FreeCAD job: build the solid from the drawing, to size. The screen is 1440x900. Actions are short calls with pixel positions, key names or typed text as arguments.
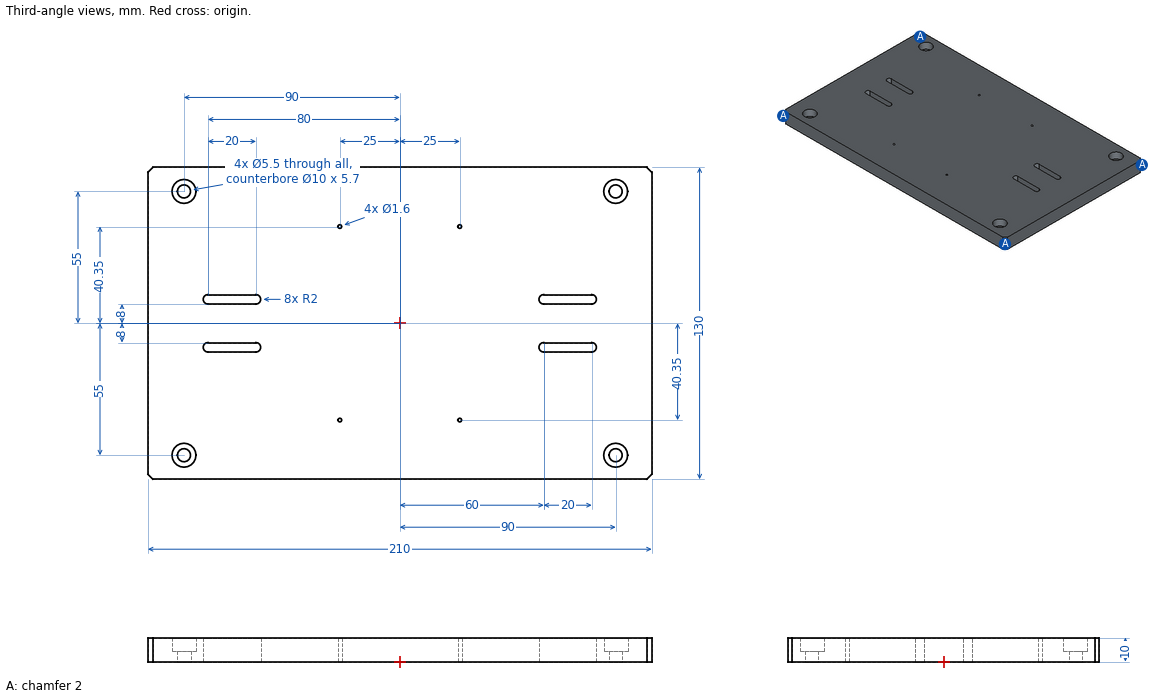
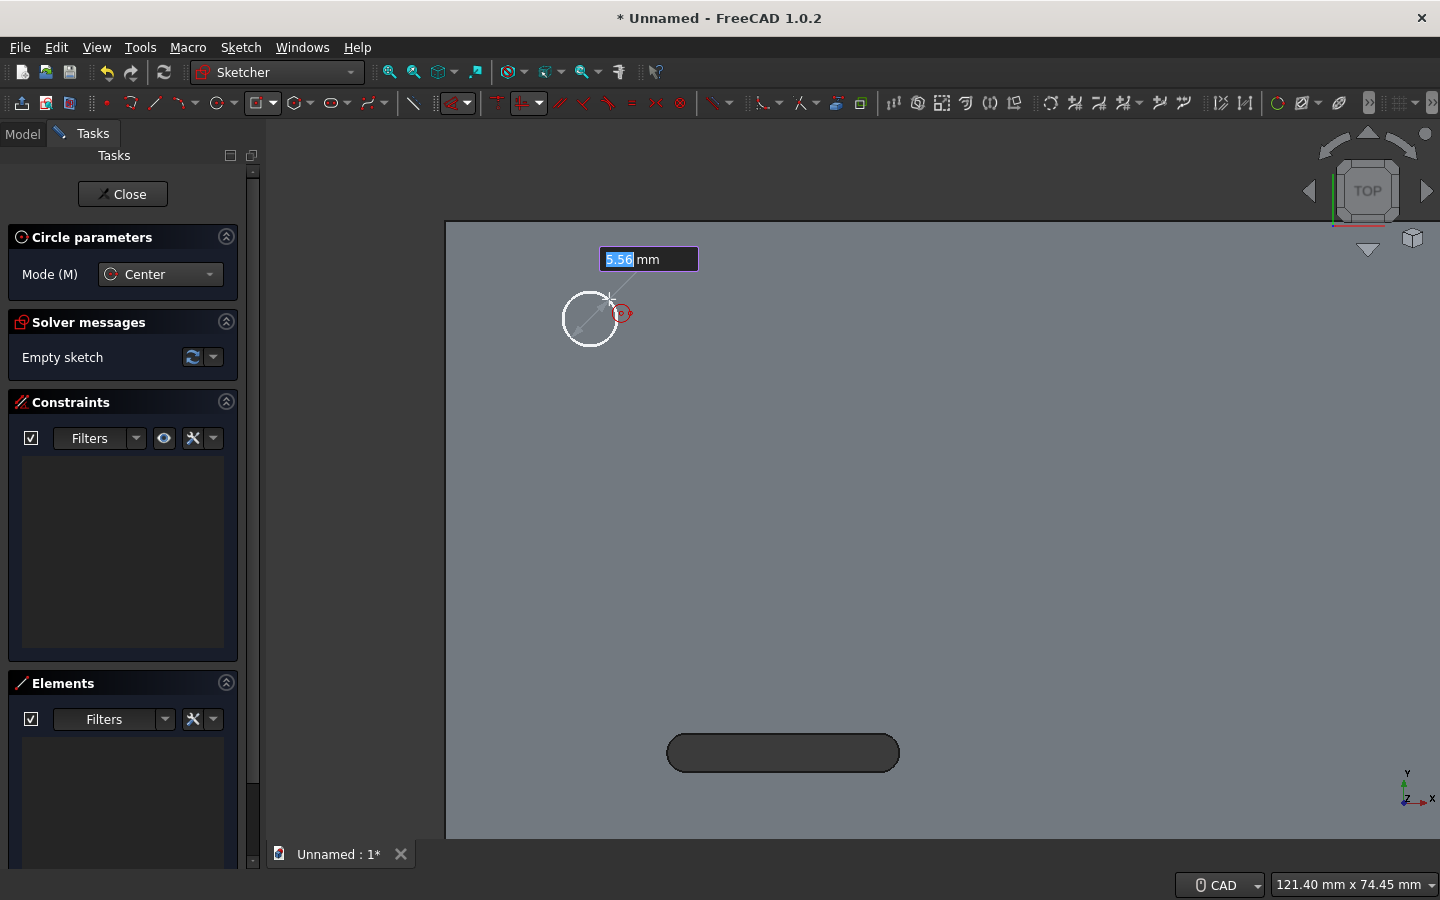
text(5.5)
key(Return)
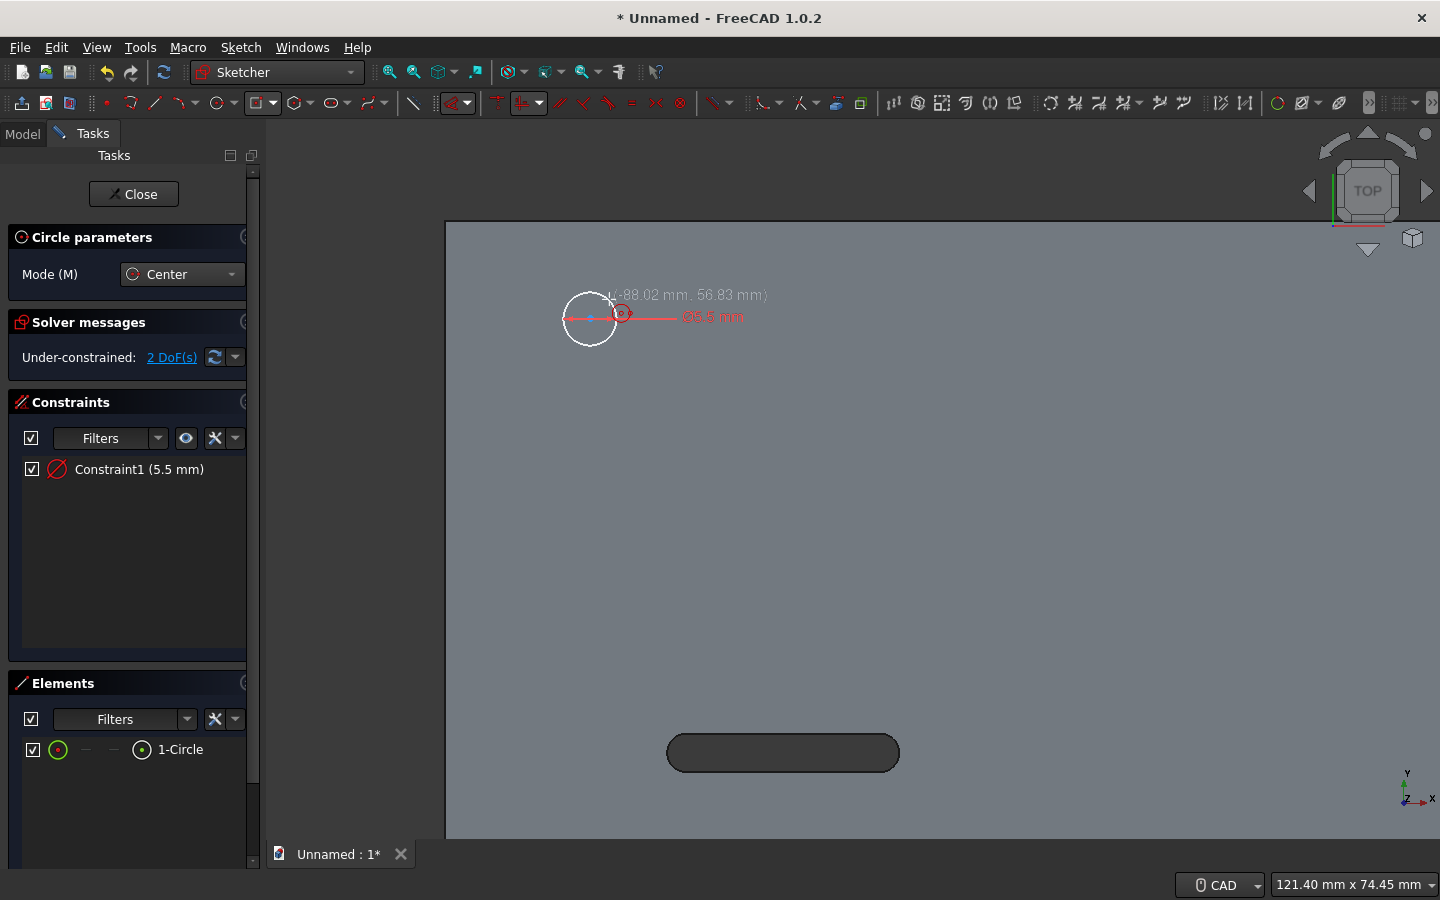
scroll(391, 263, down, 5)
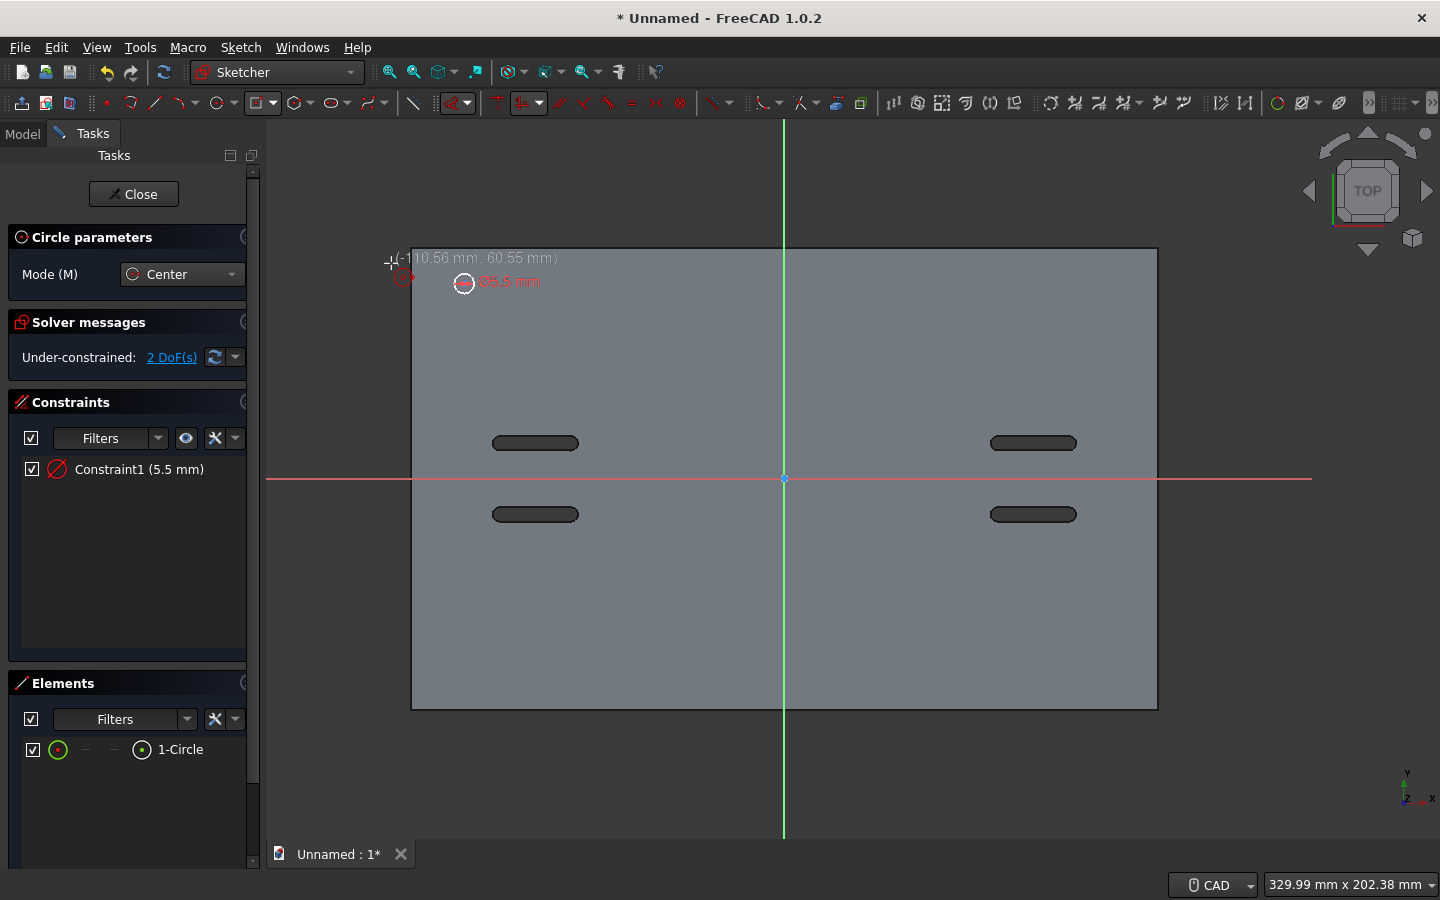
scroll(464, 675, up, 5)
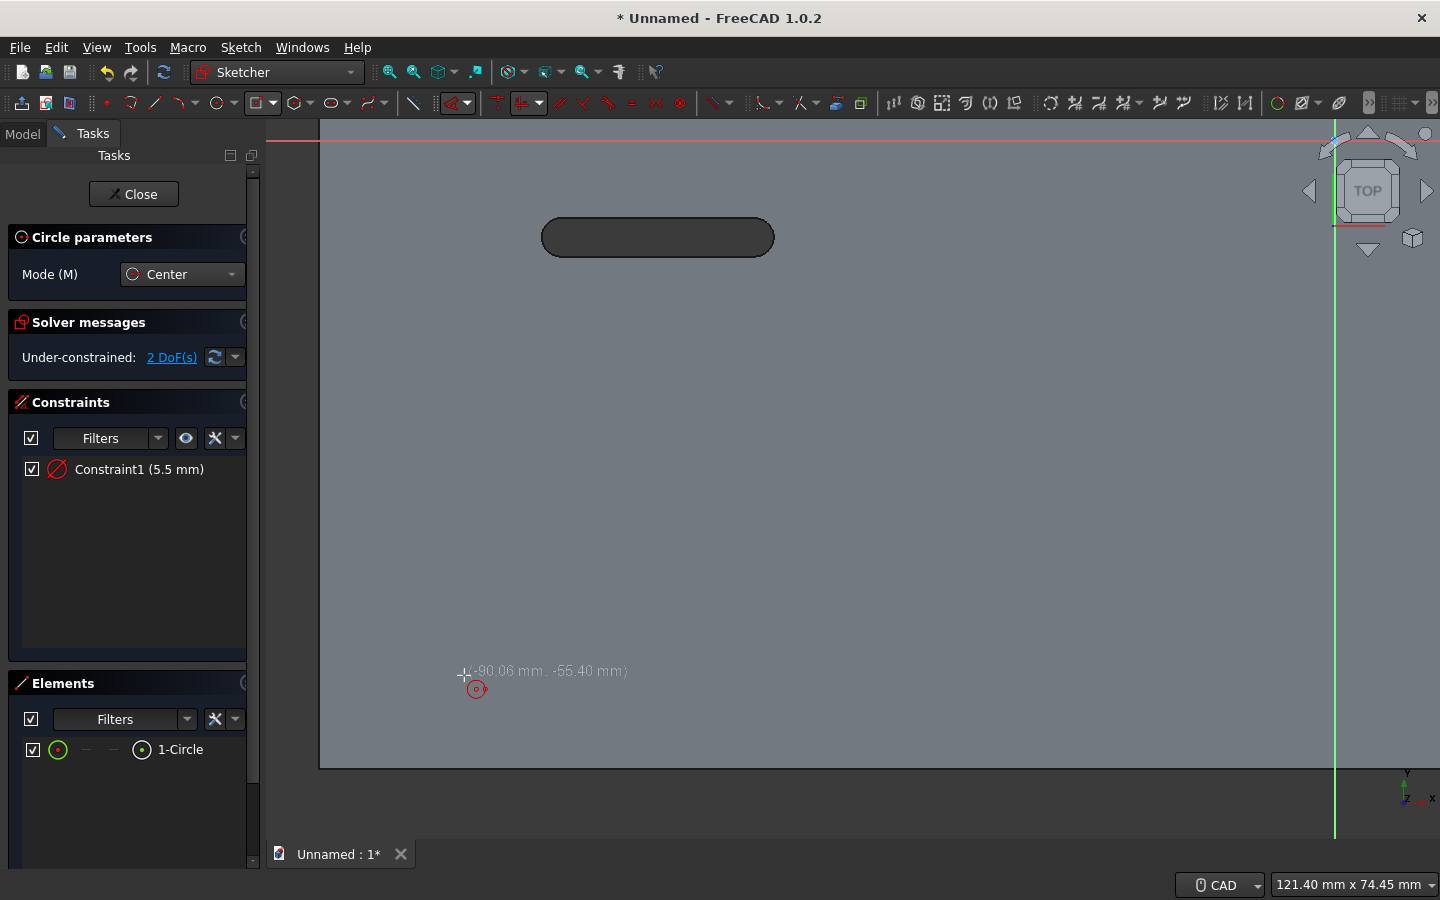
click(464, 673)
move(483, 654)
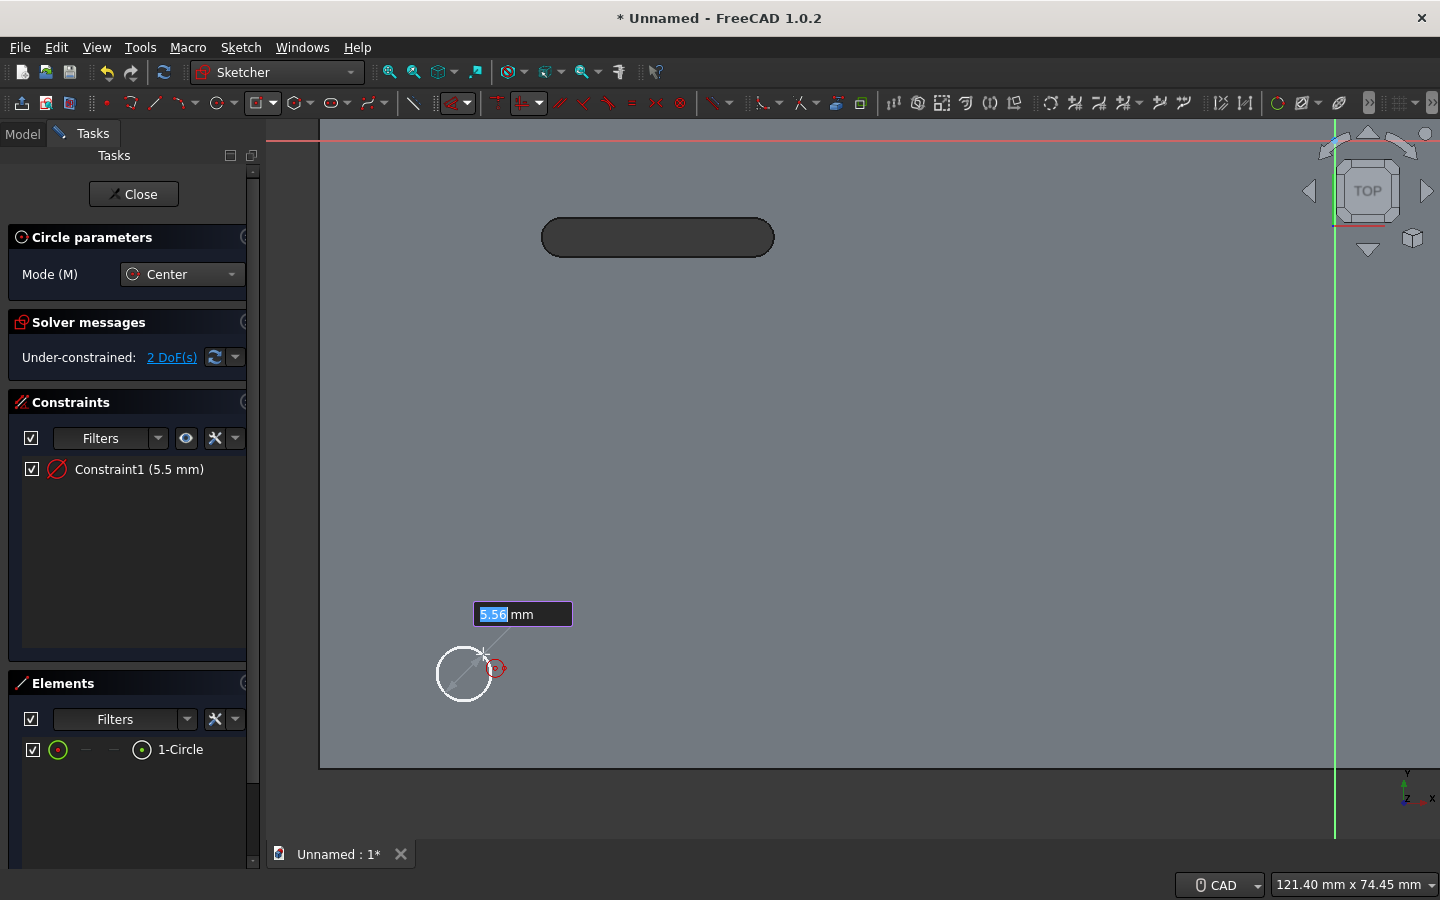
text(5.5)
key(Return)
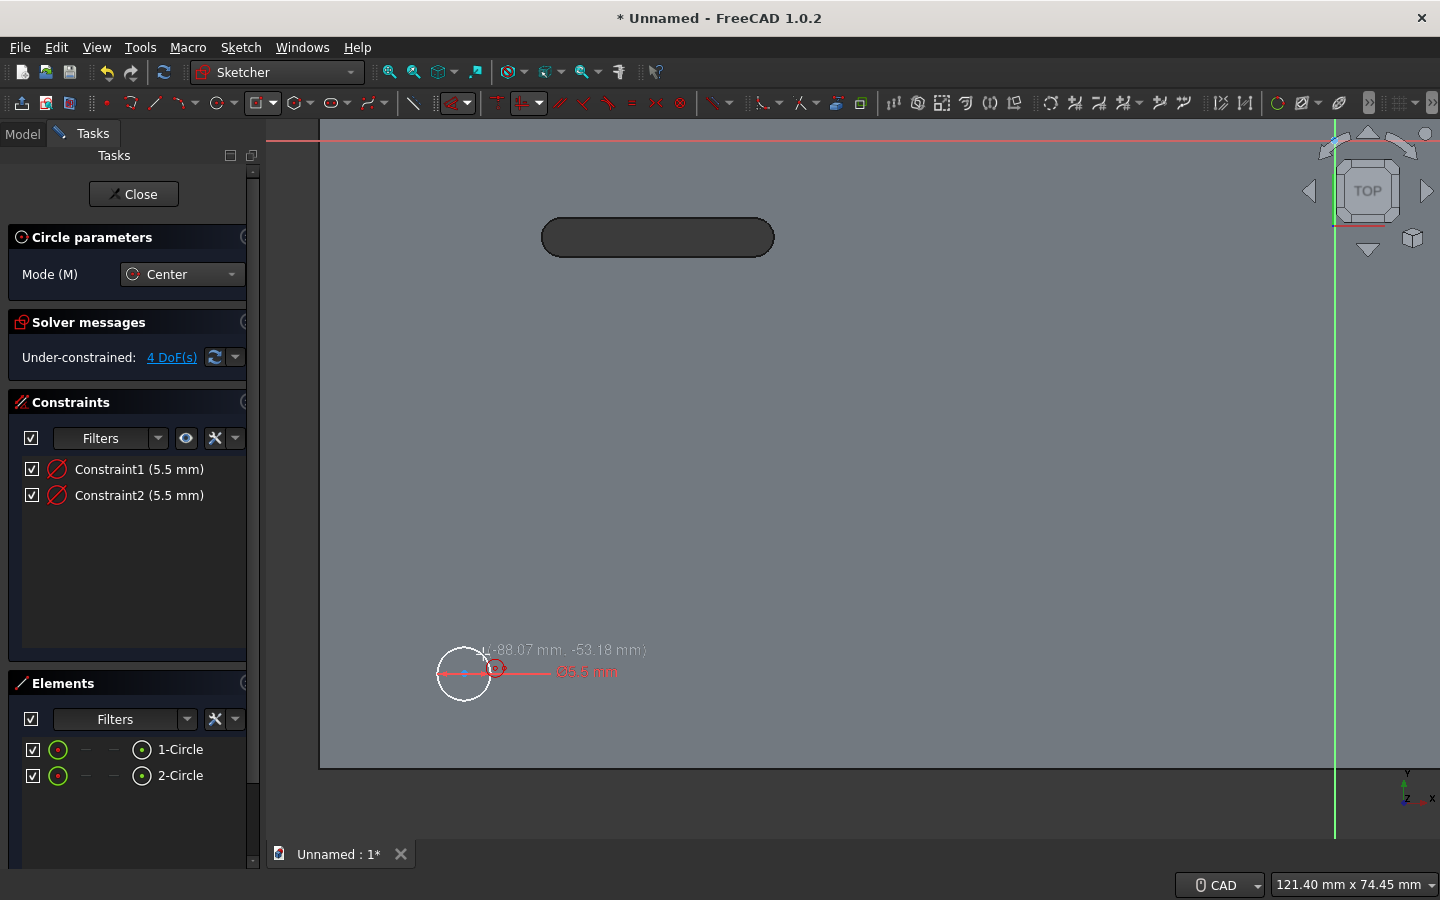
scroll(464, 676, down, 5)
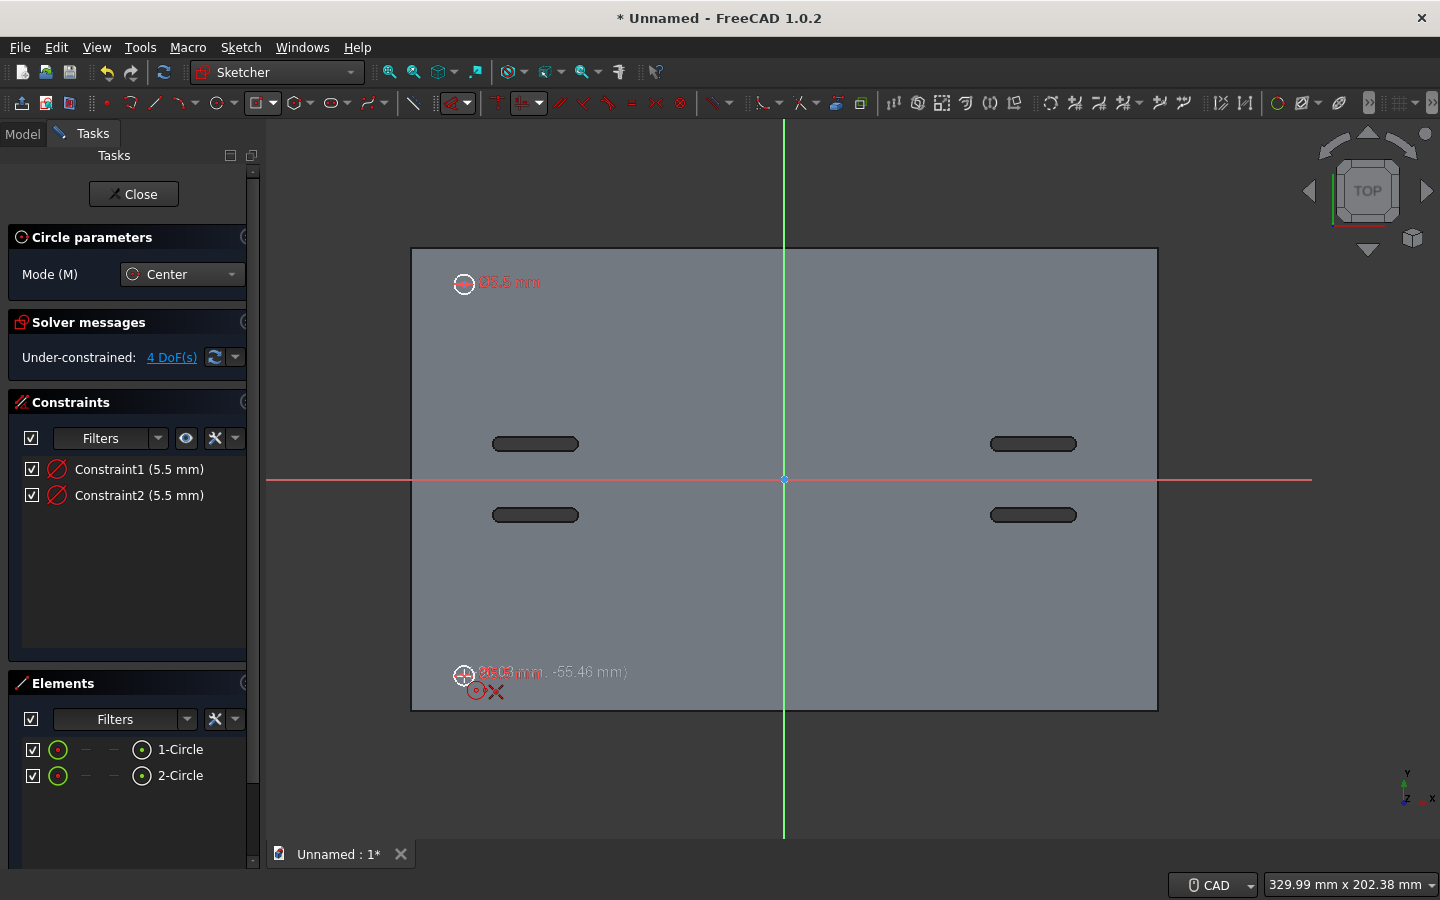
scroll(1105, 675, up, 5)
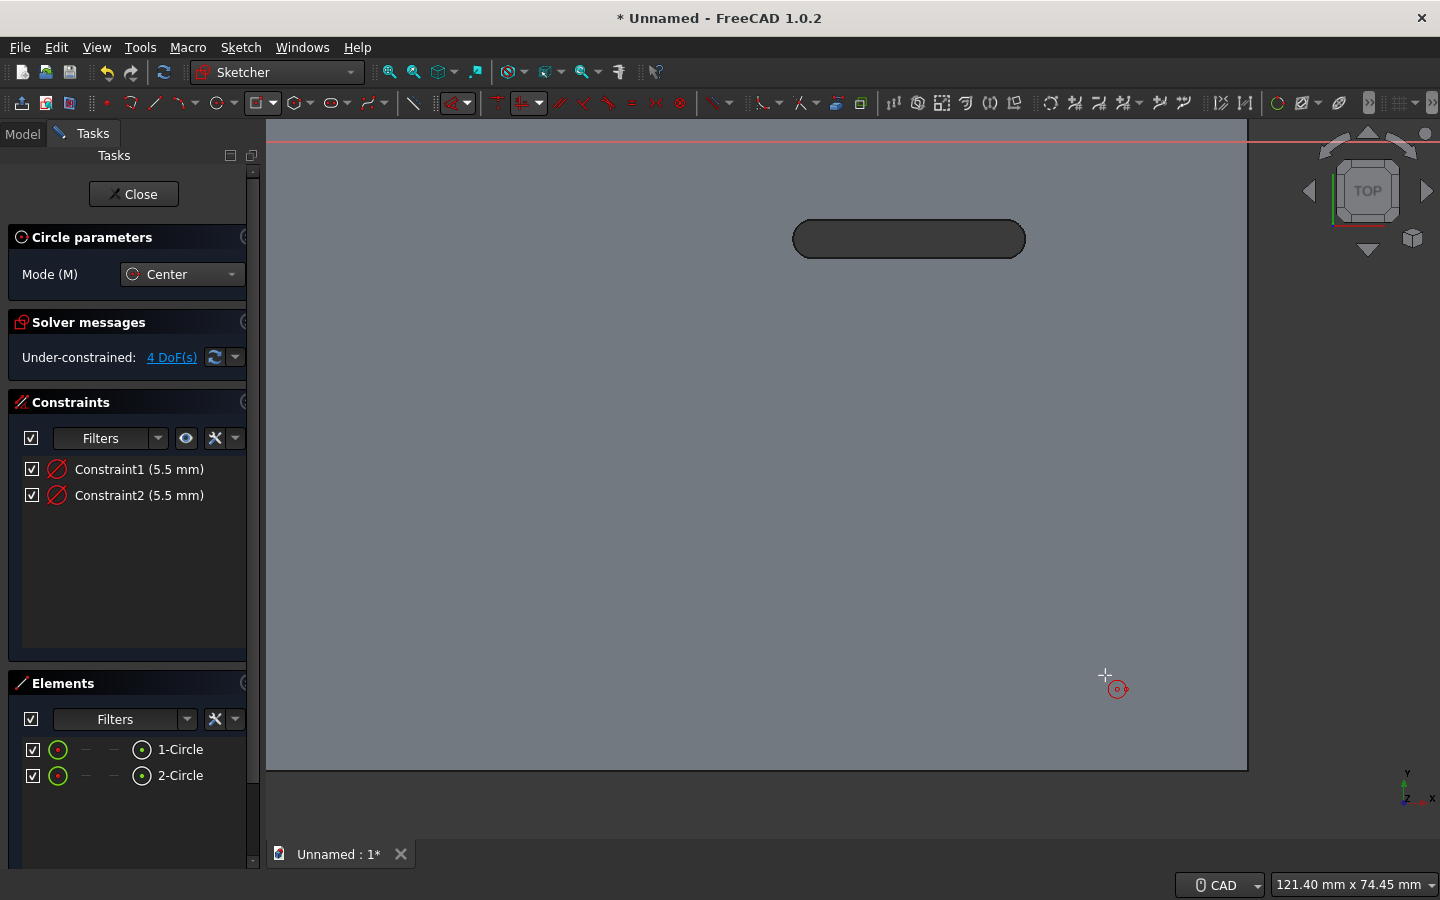
click(1103, 674)
move(1122, 655)